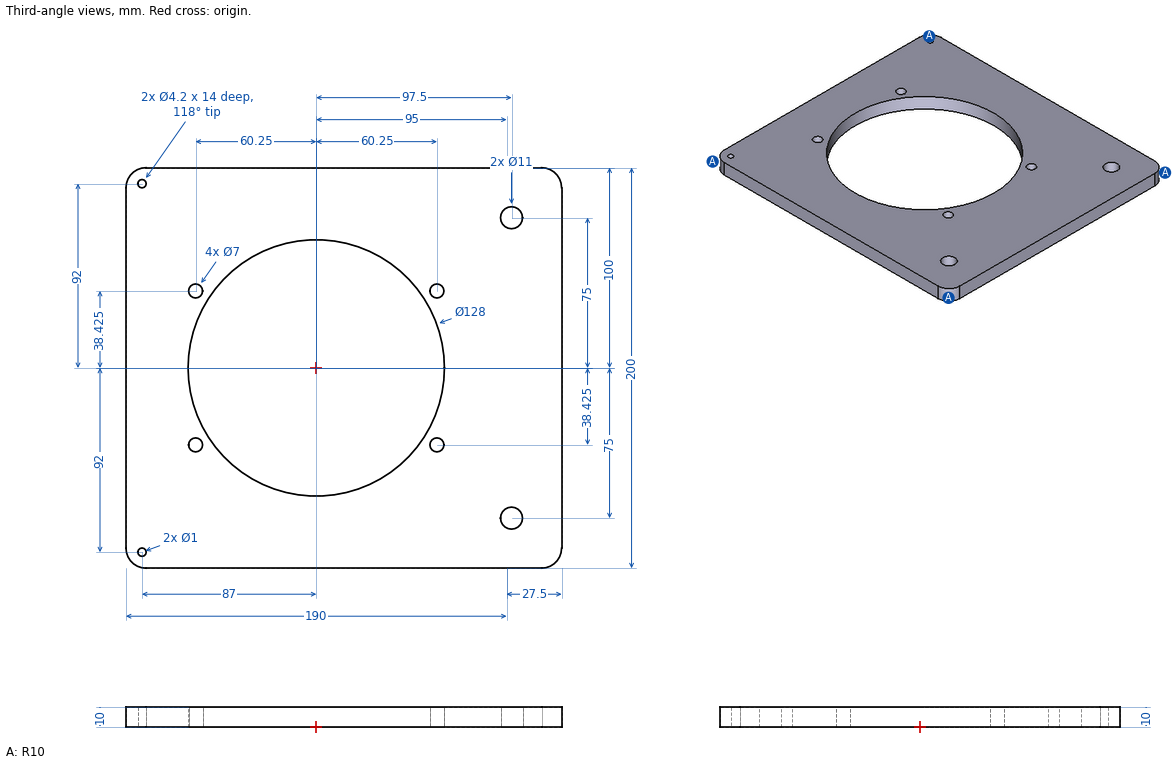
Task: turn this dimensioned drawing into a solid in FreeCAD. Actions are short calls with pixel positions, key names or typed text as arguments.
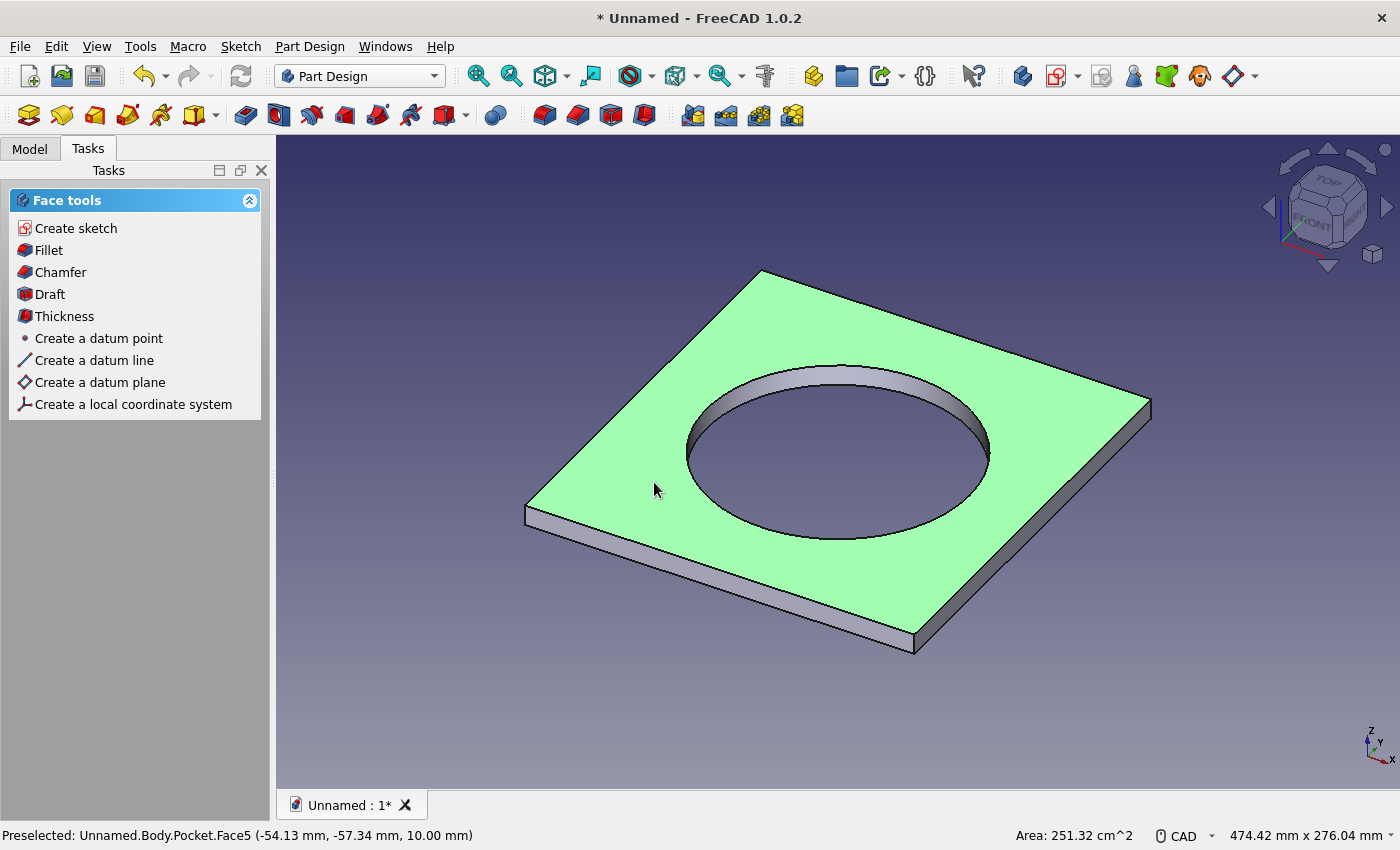
click(1056, 76)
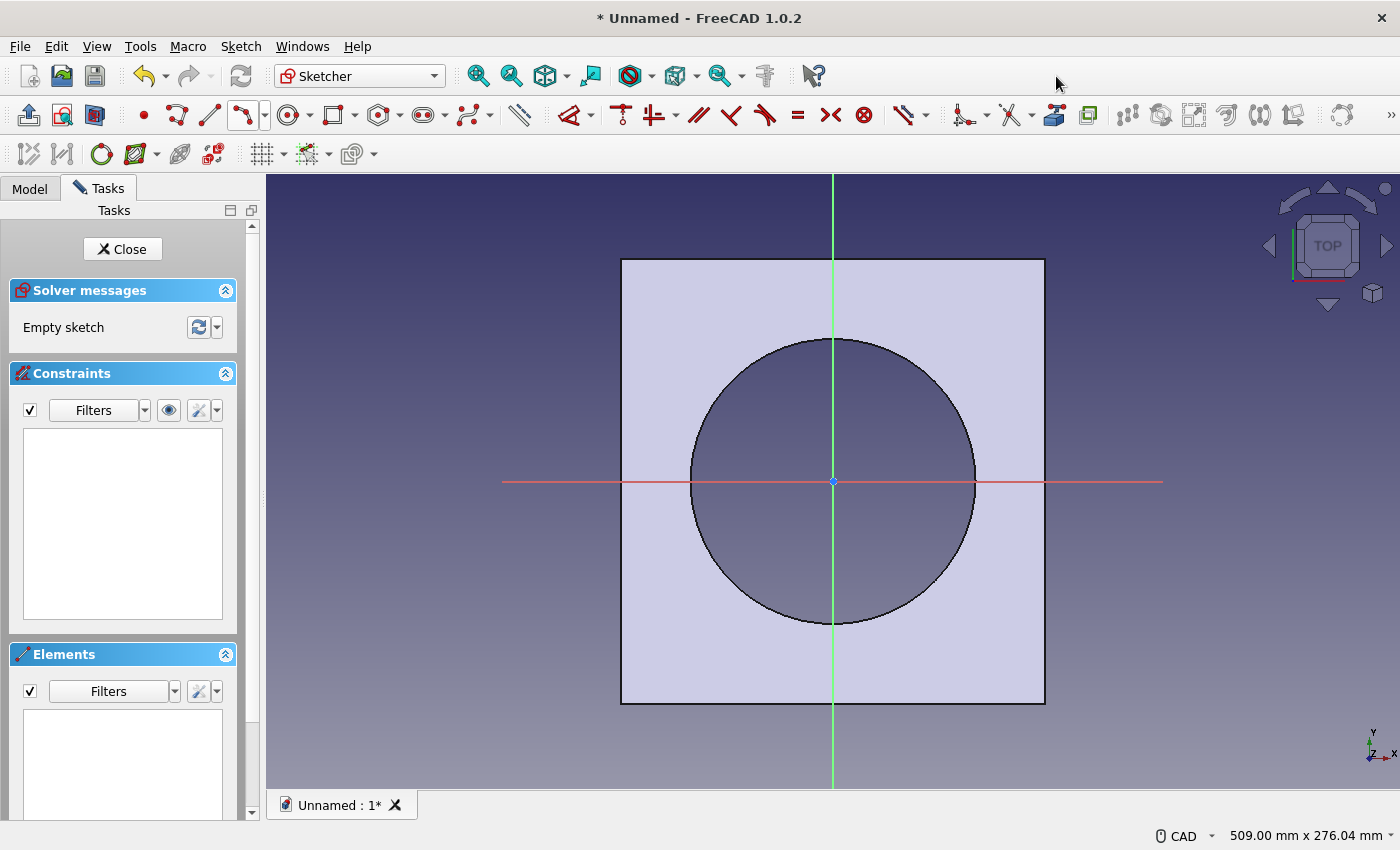
scroll(889, 482, up, 4)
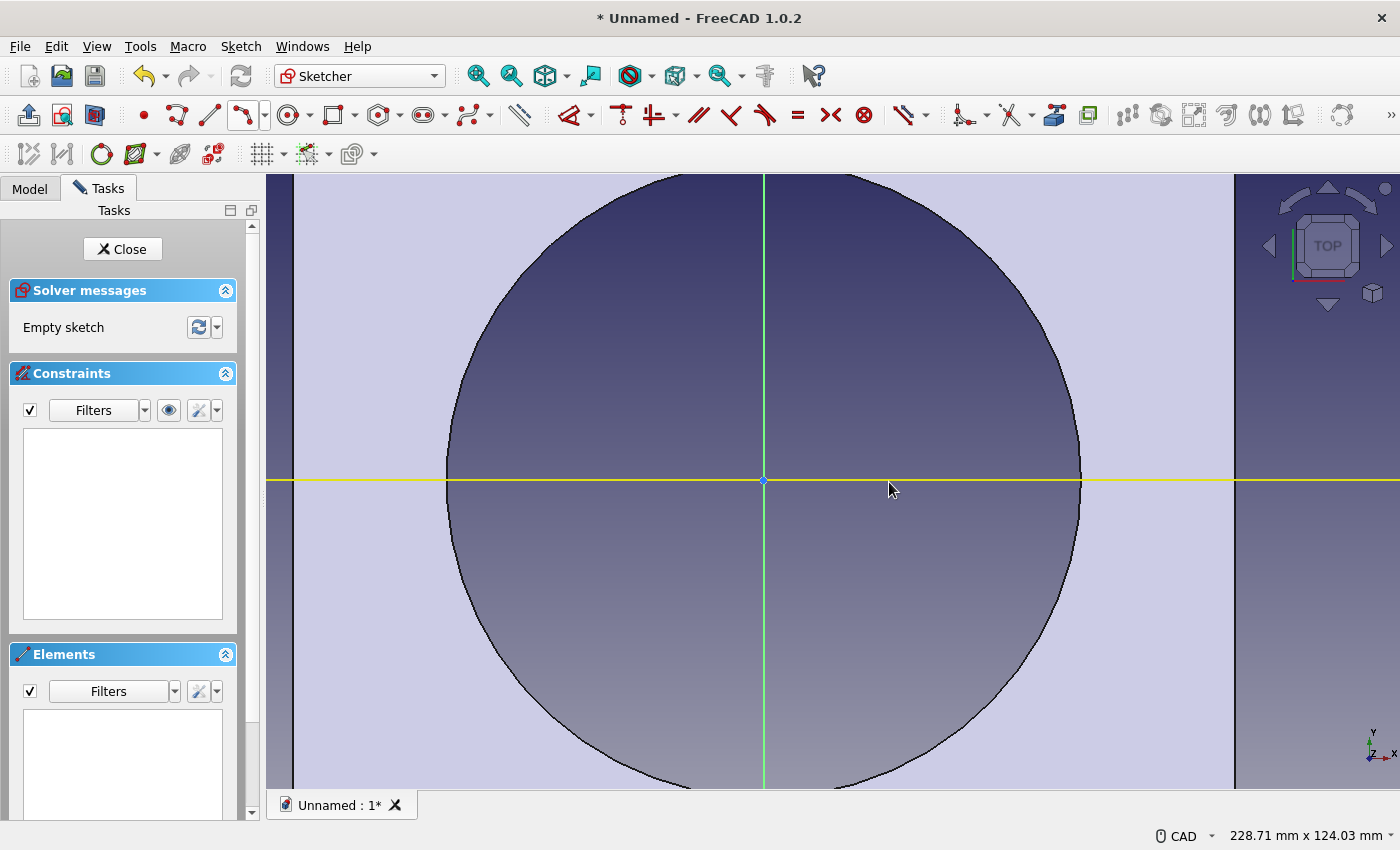
key(g)
key(c)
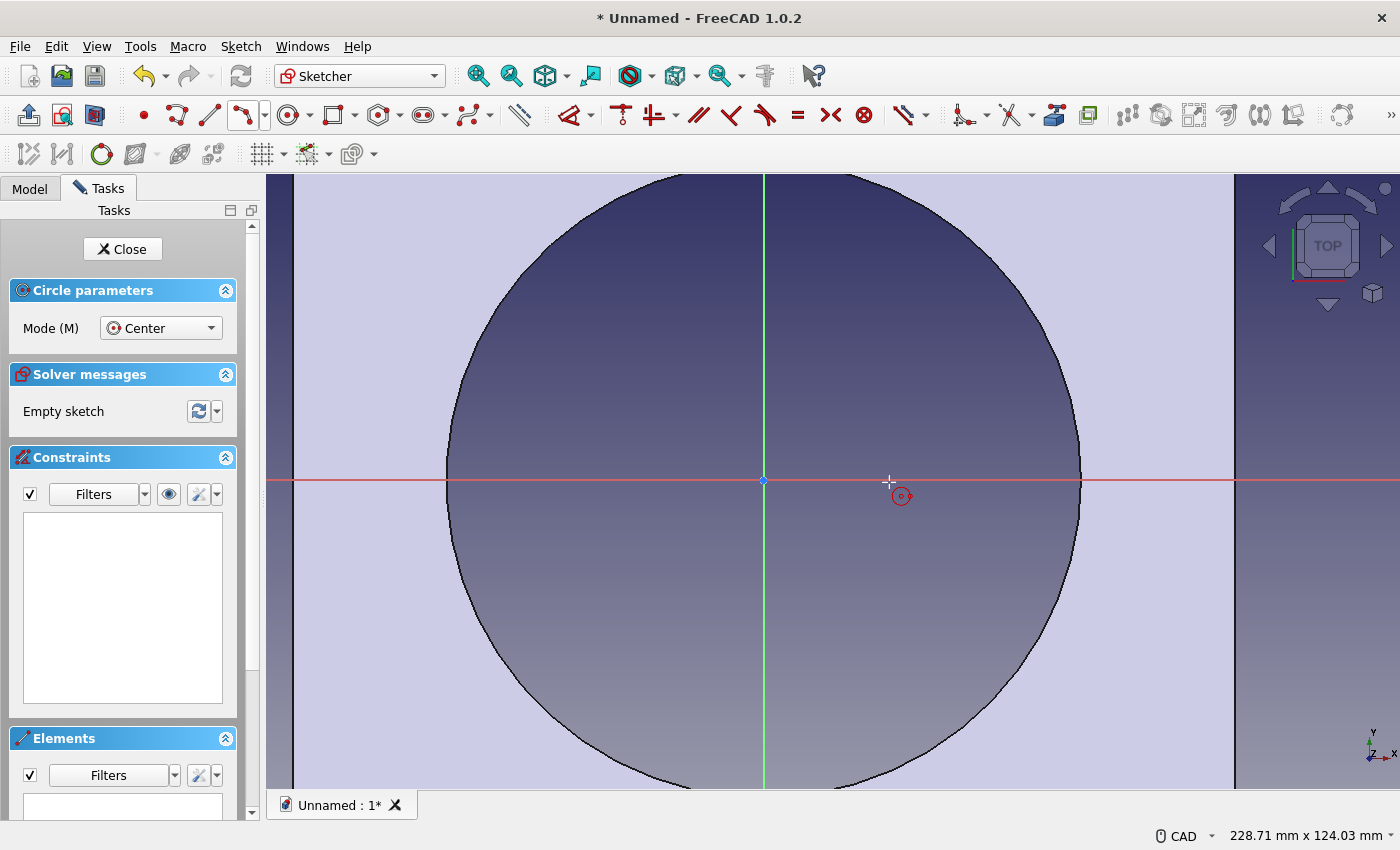
scroll(465, 290, up, 2)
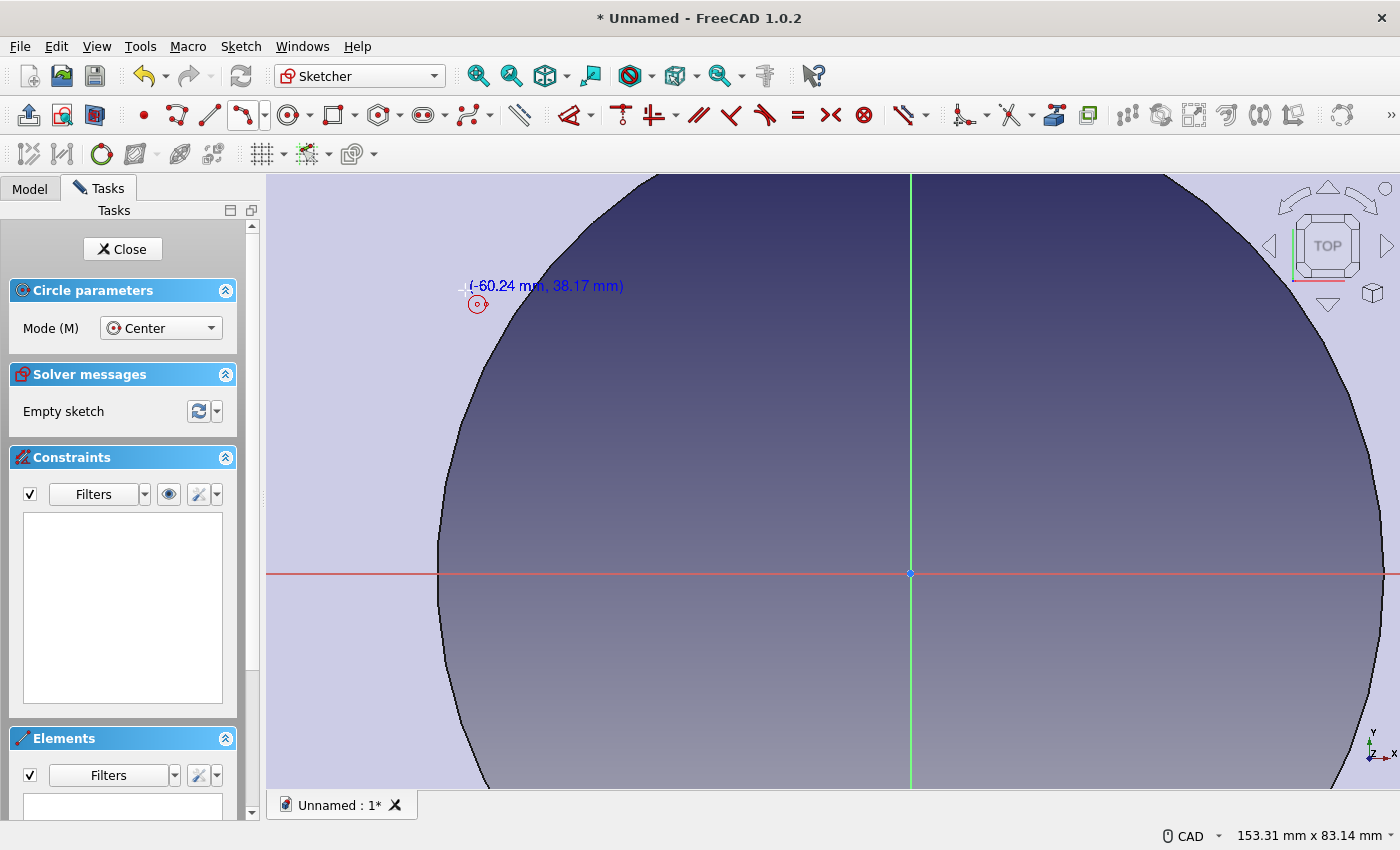
click(465, 290)
move(483, 271)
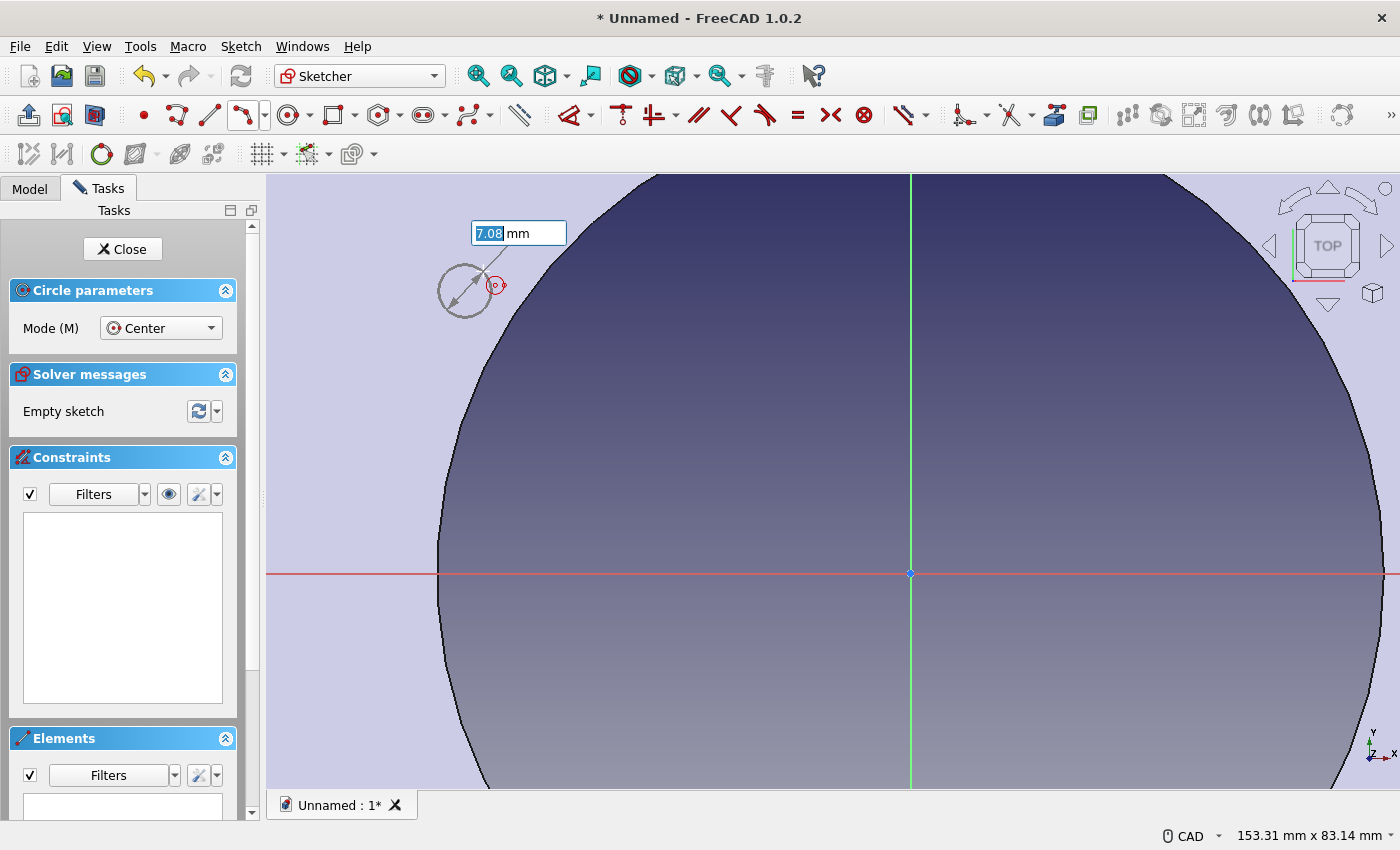
text(7)
key(Return)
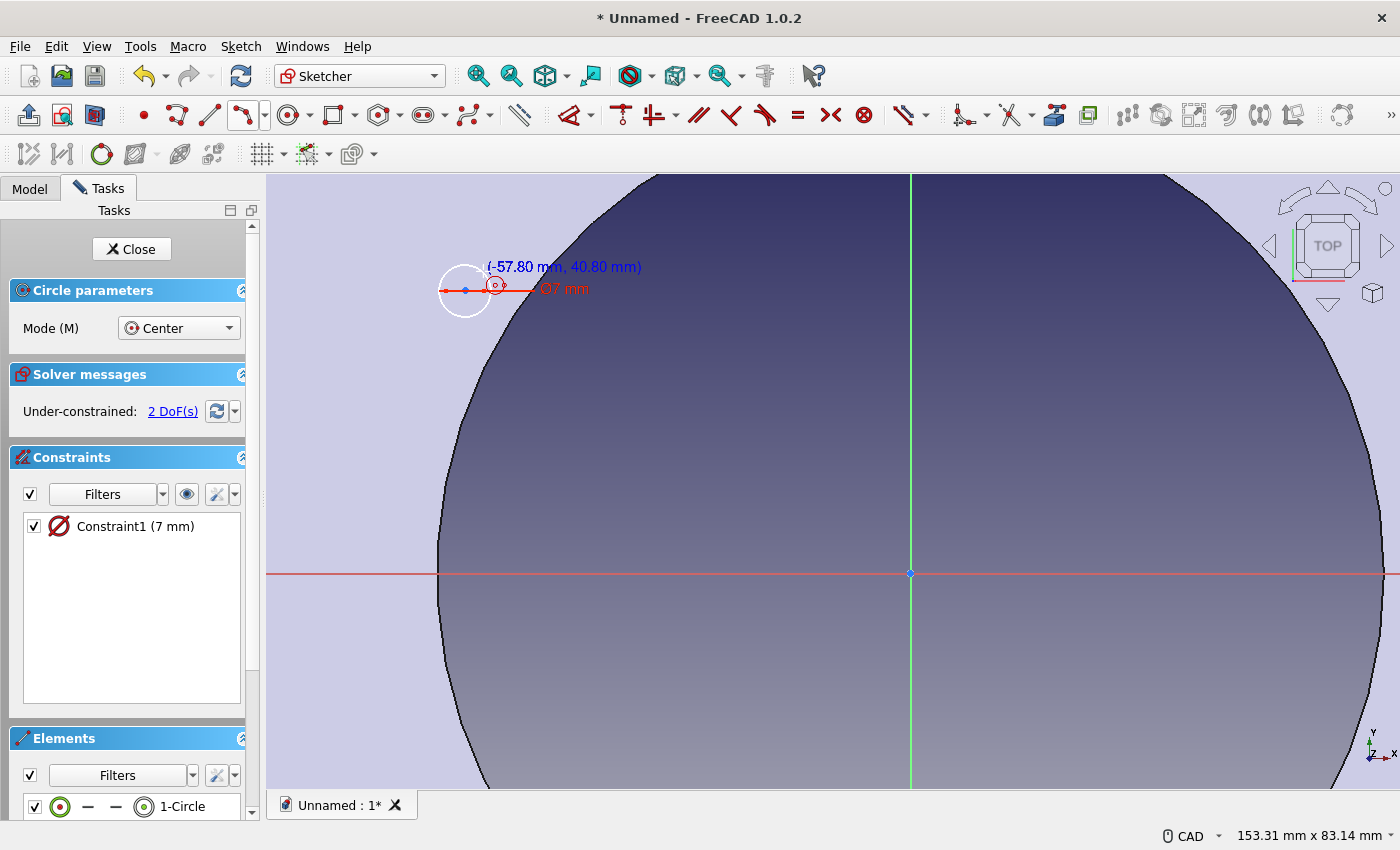
scroll(468, 294, down, 2)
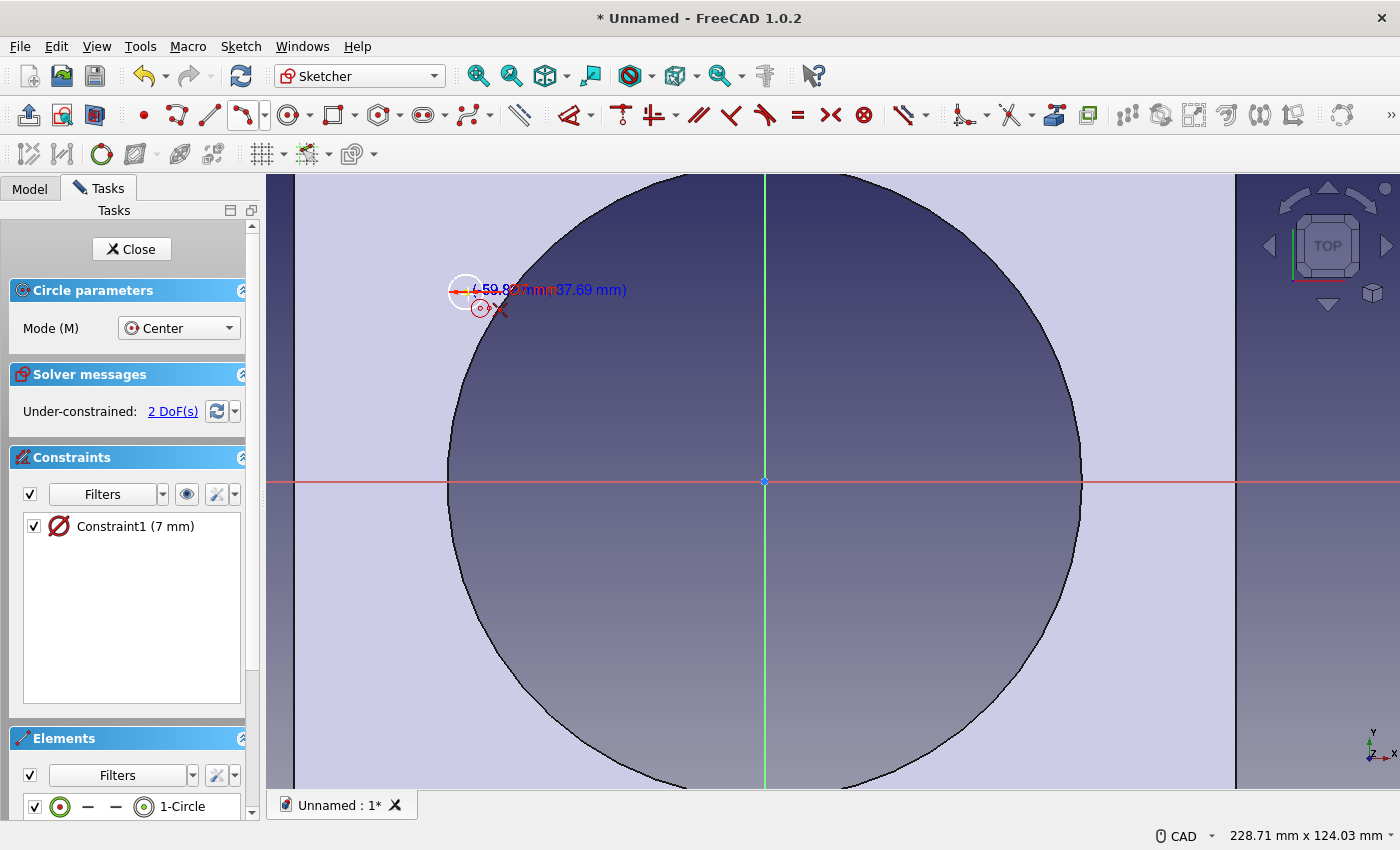
scroll(1063, 291, up, 2)